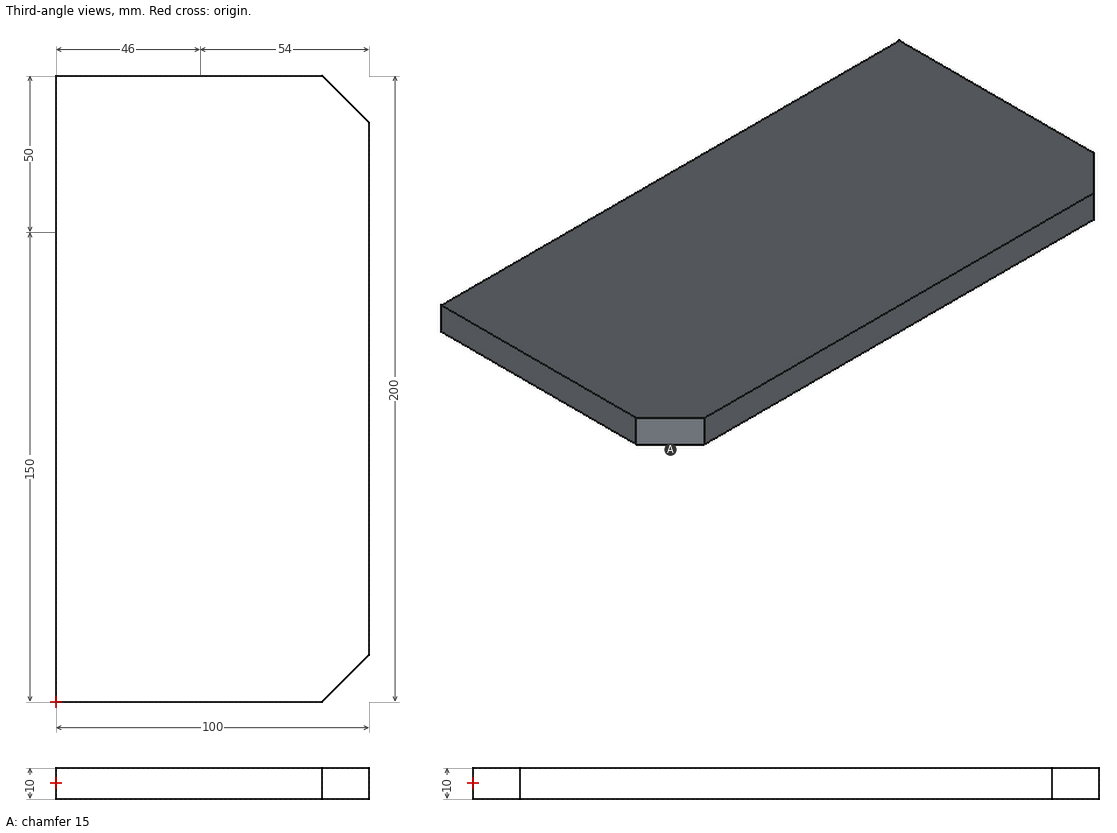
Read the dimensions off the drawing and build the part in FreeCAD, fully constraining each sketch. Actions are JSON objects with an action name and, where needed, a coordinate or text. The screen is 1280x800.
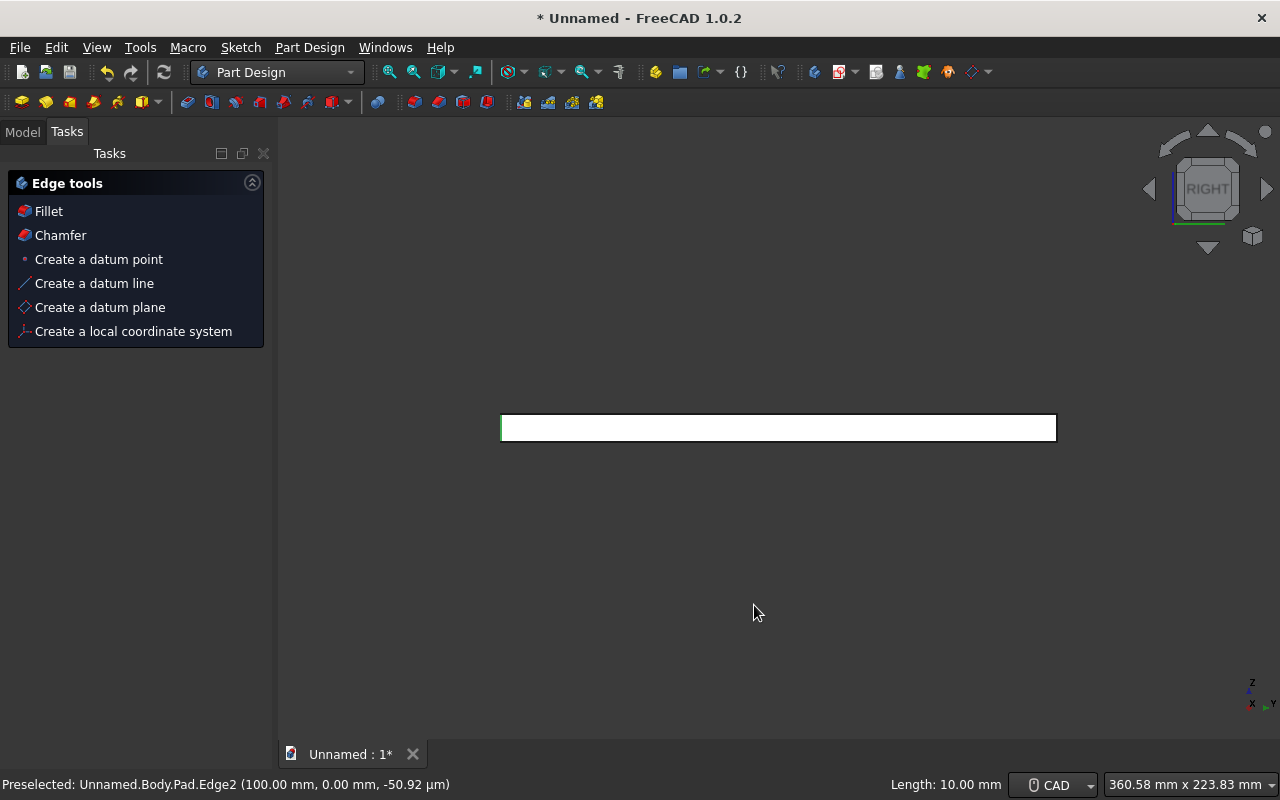
{"action": "left_click", "coordinate": [1057, 427], "text": "ctrl"}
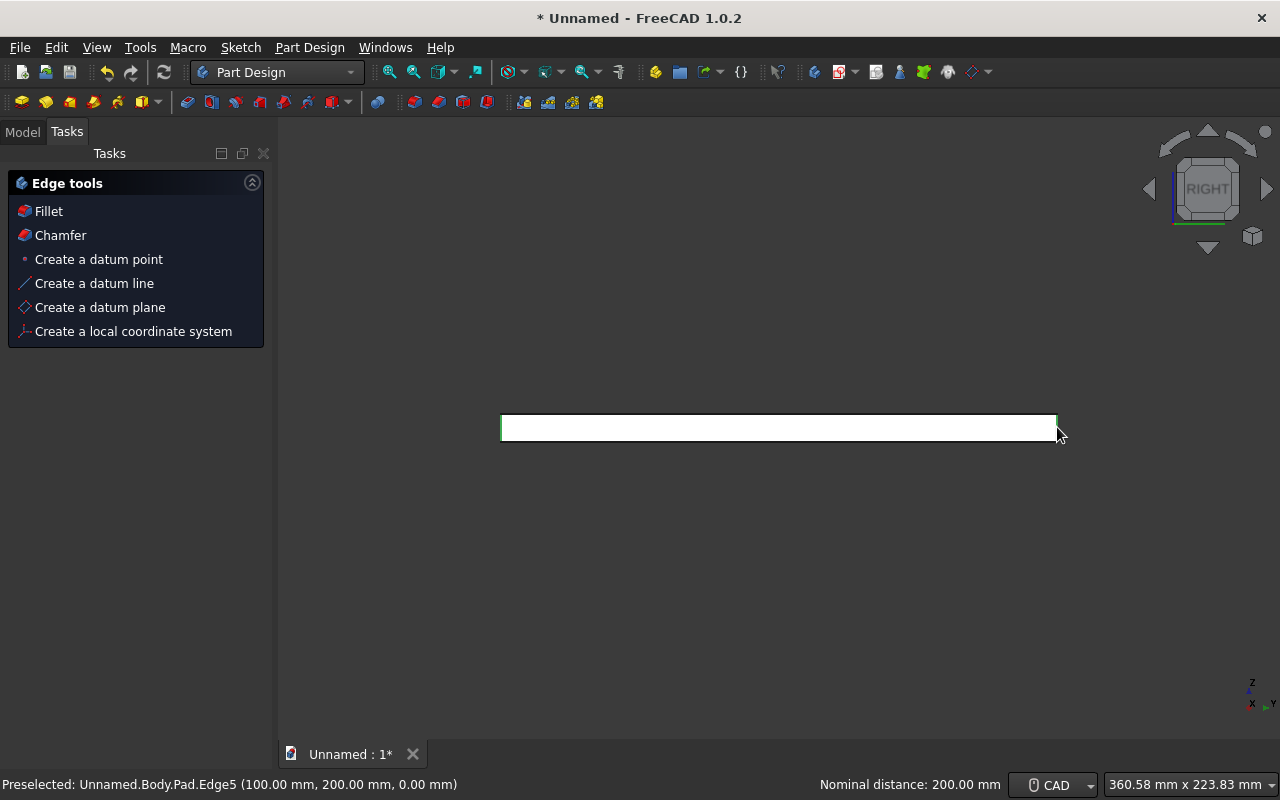
{"action": "left_click", "coordinate": [440, 102]}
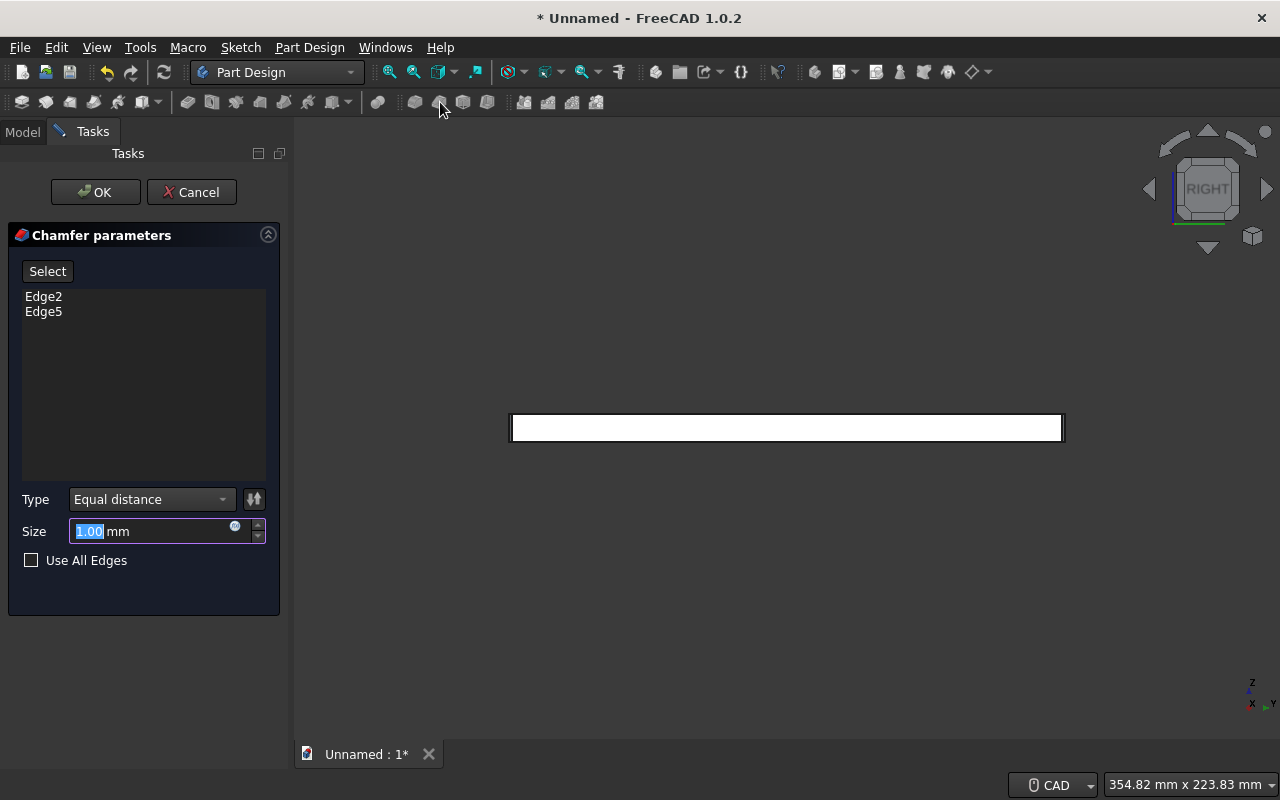
{"action": "type", "text": "15"}
{"action": "key", "text": "Tab"}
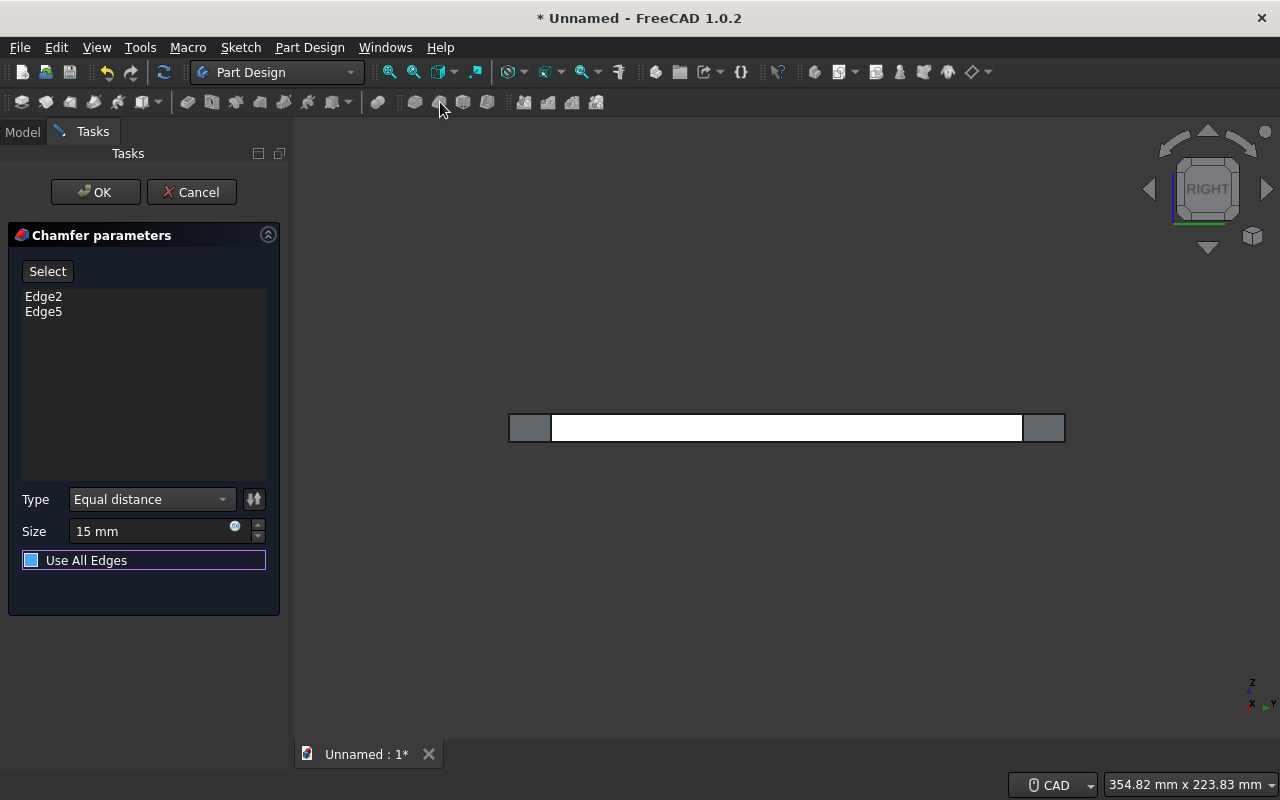
{"action": "left_click", "coordinate": [96, 192]}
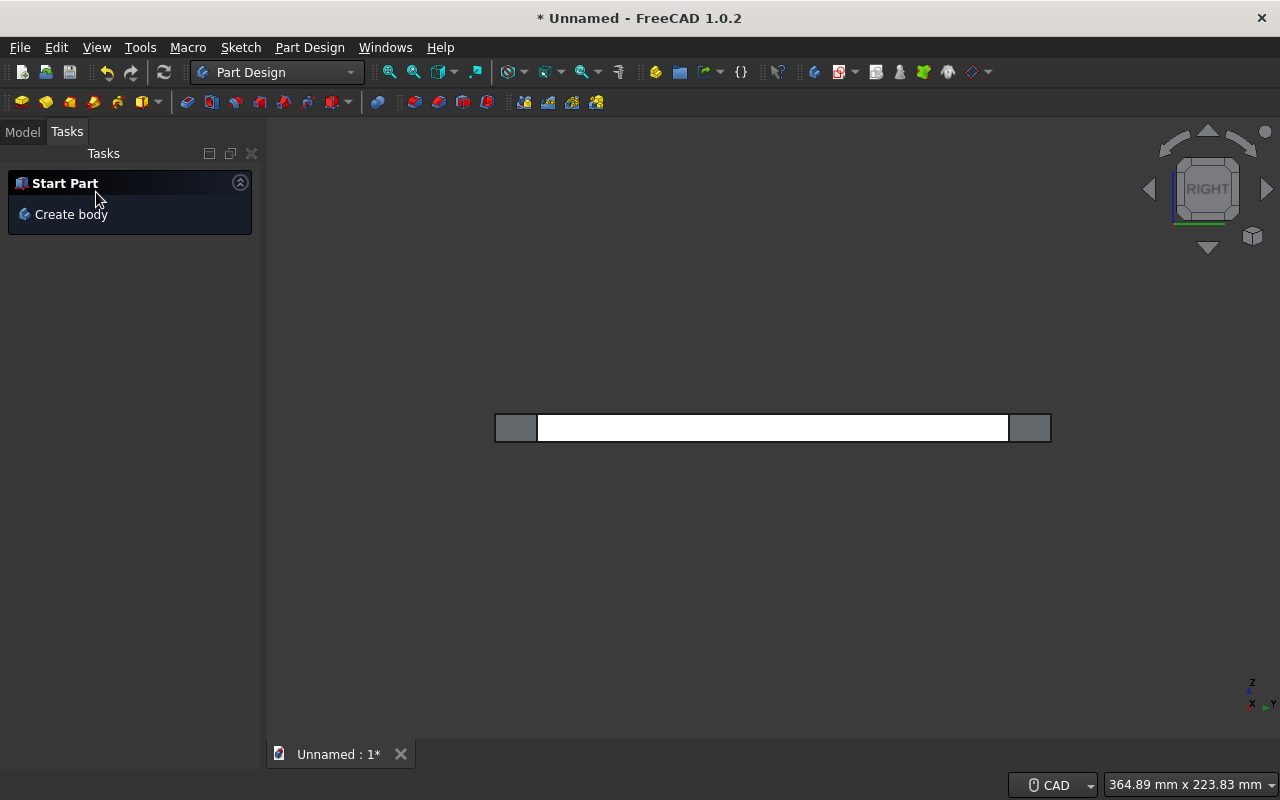
{"action": "key", "text": "0"}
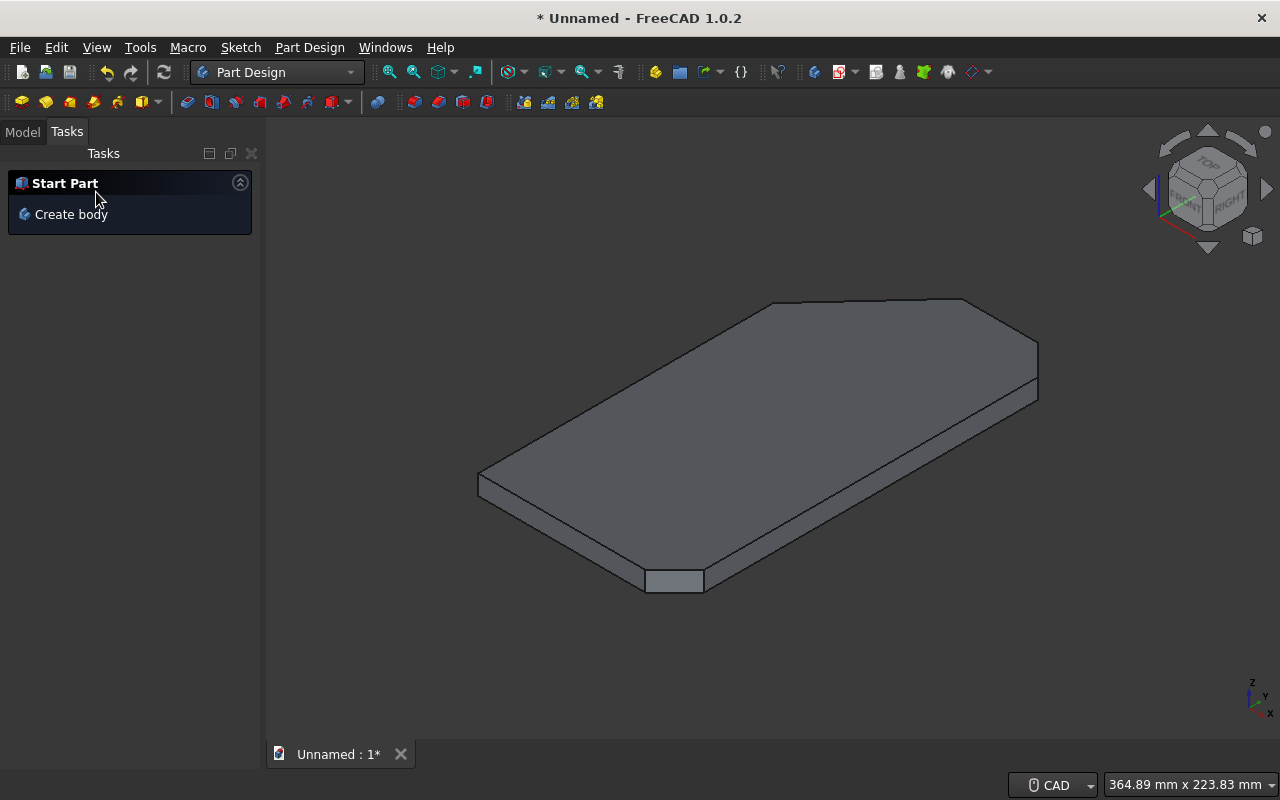
{"action": "left_click", "coordinate": [829, 383]}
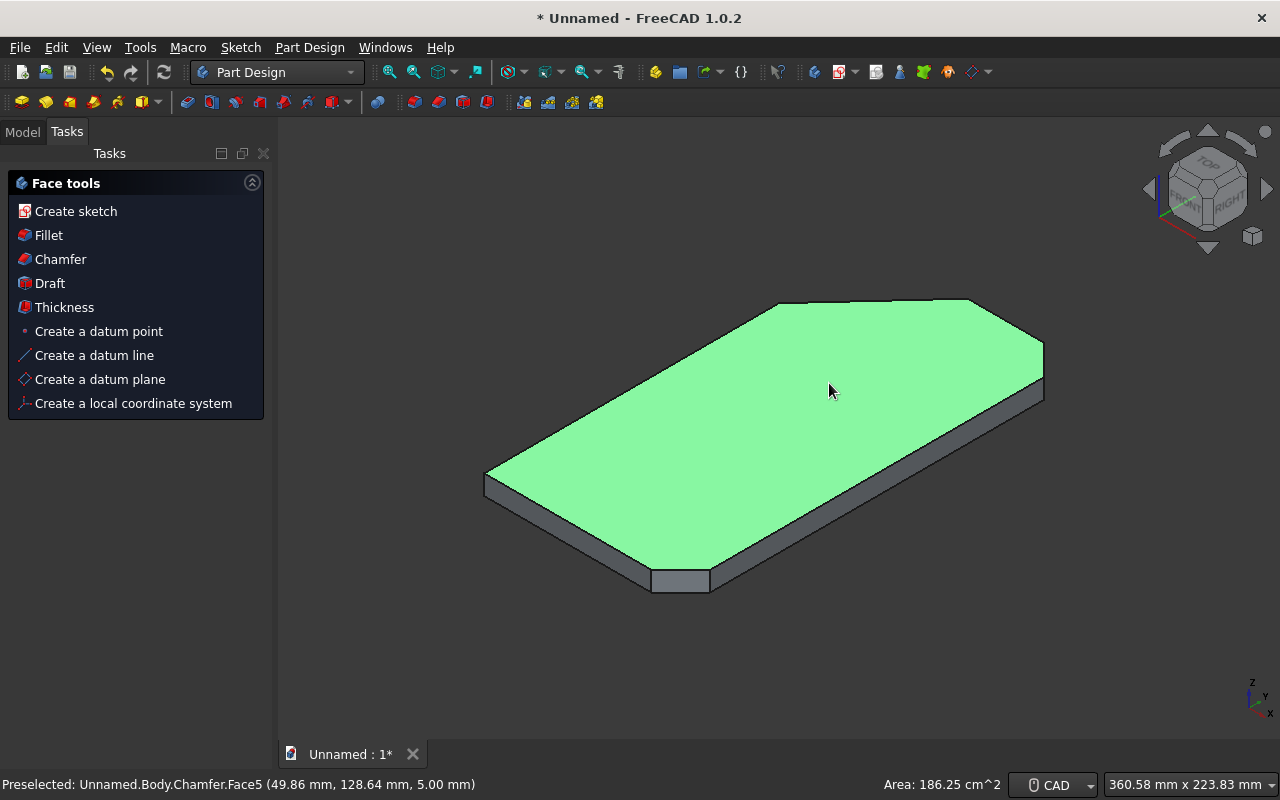
{"action": "left_click", "coordinate": [840, 72]}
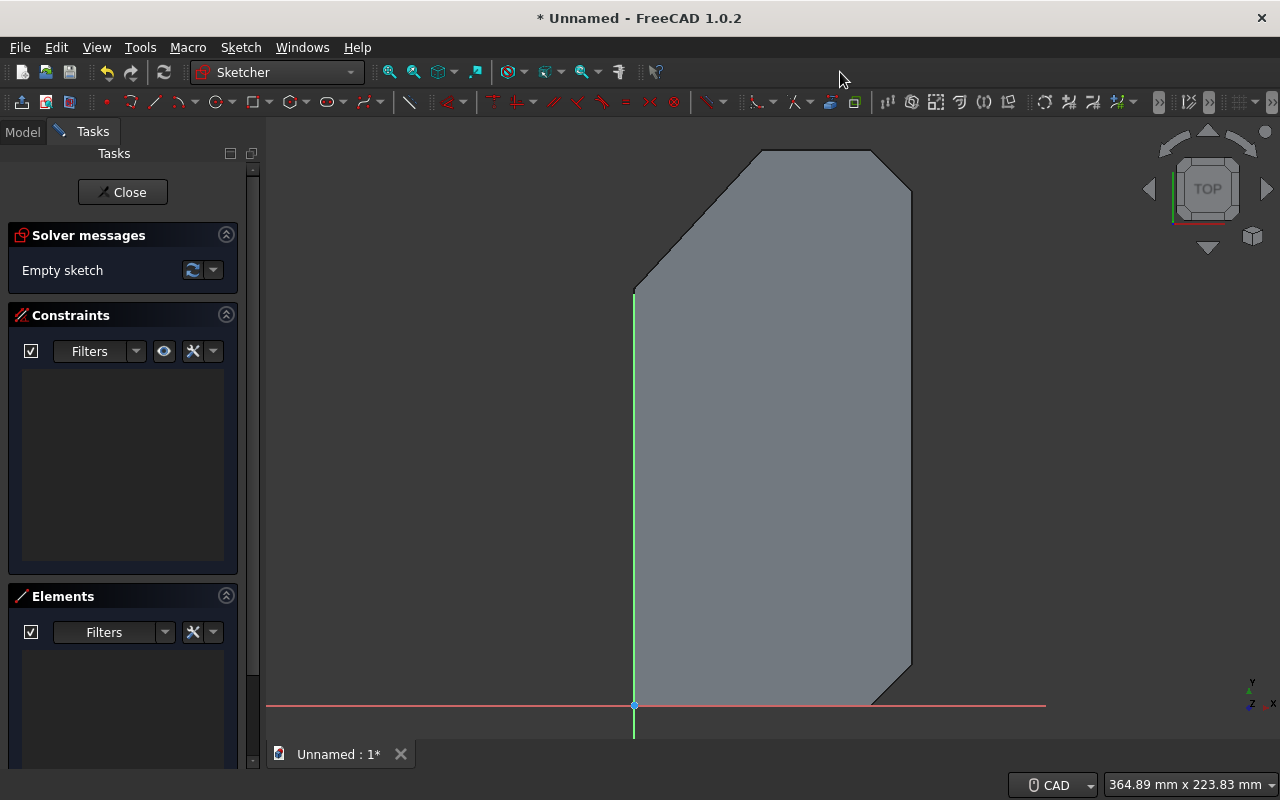
{"action": "scroll", "coordinate": [704, 428], "scroll_direction": "down", "scroll_amount": 5}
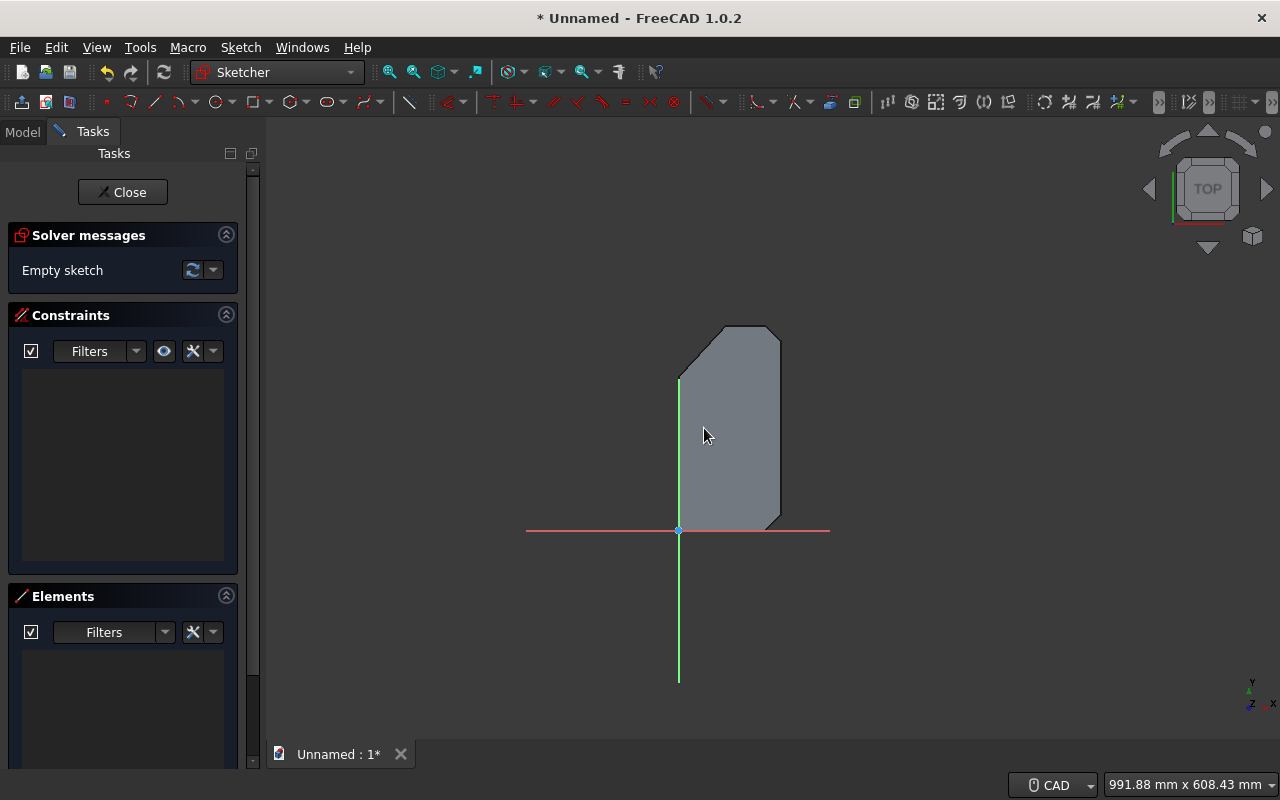
{"action": "scroll", "coordinate": [702, 340], "scroll_direction": "up", "scroll_amount": 10}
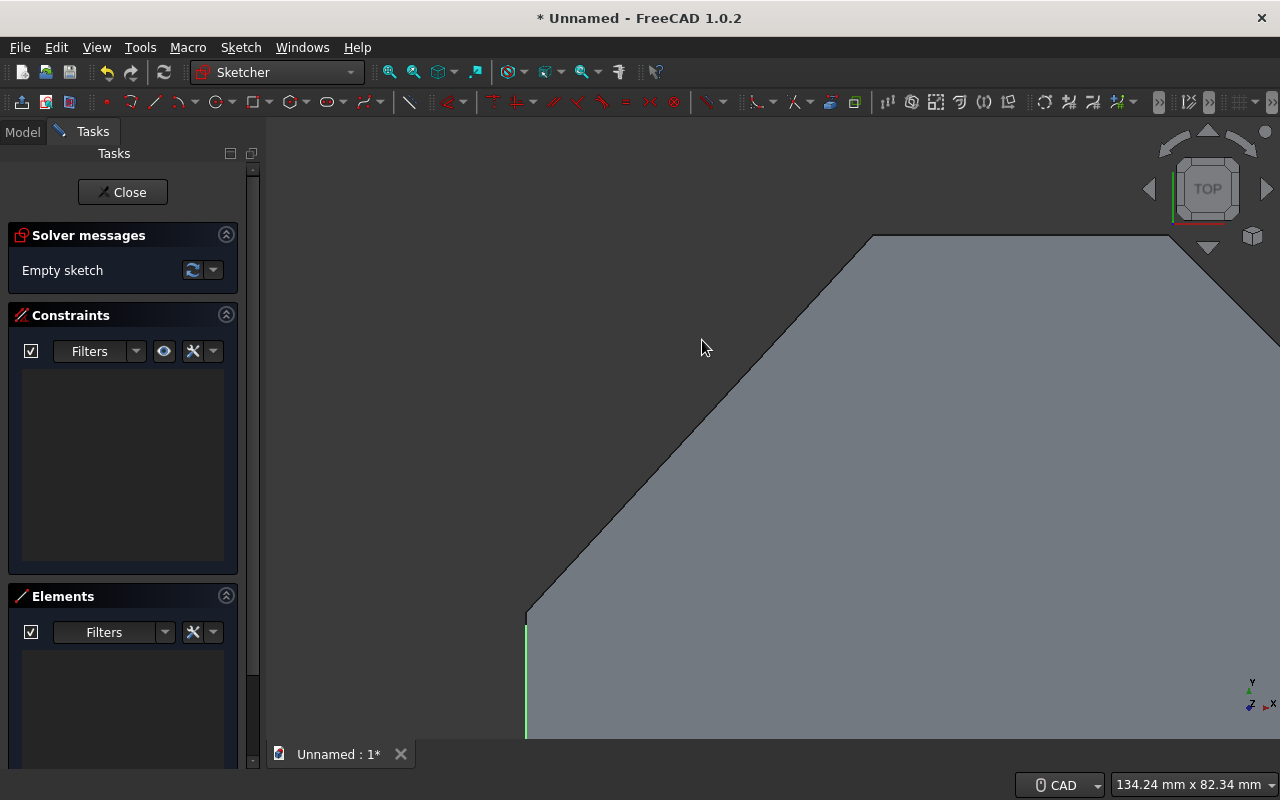
{"action": "left_click", "coordinate": [132, 102]}